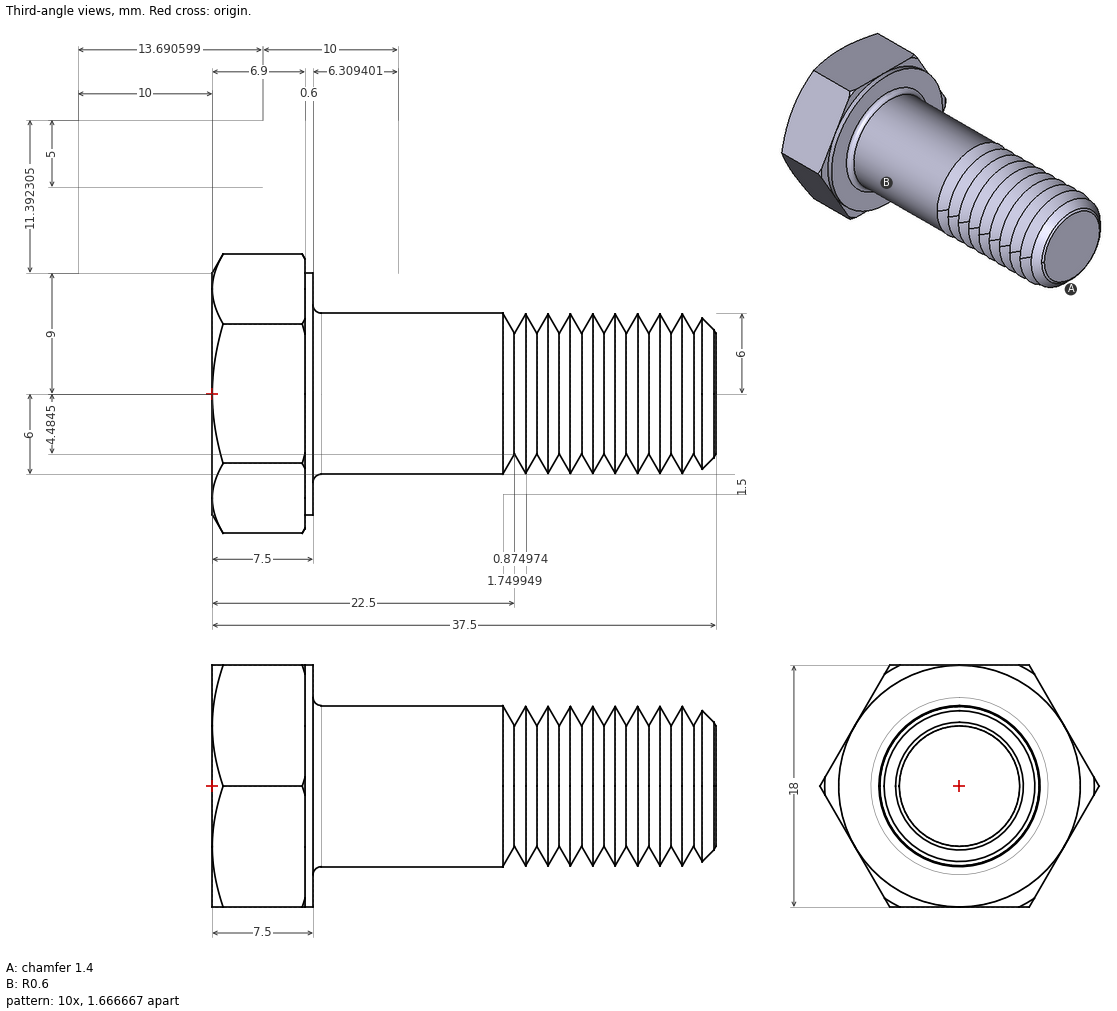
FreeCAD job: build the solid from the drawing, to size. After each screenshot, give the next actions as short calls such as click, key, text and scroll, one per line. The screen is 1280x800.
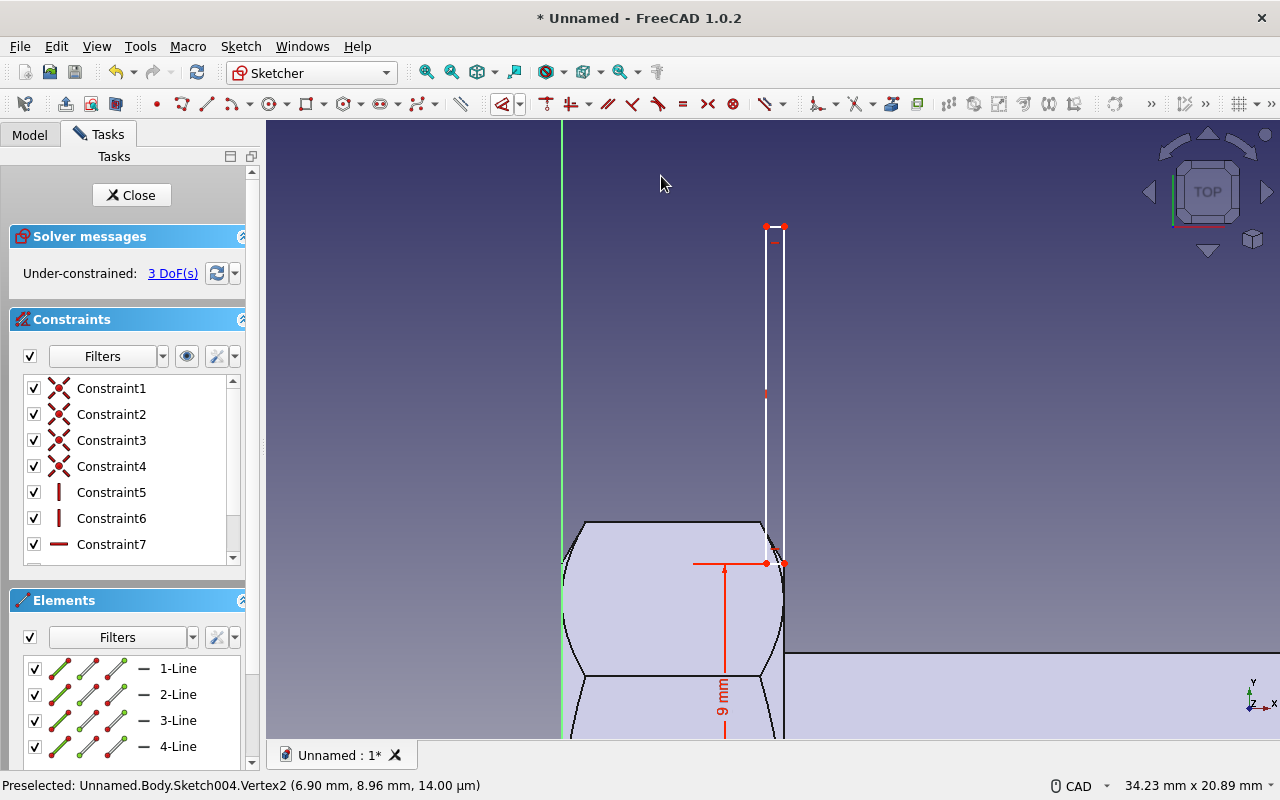
scroll(775, 564, up, 5)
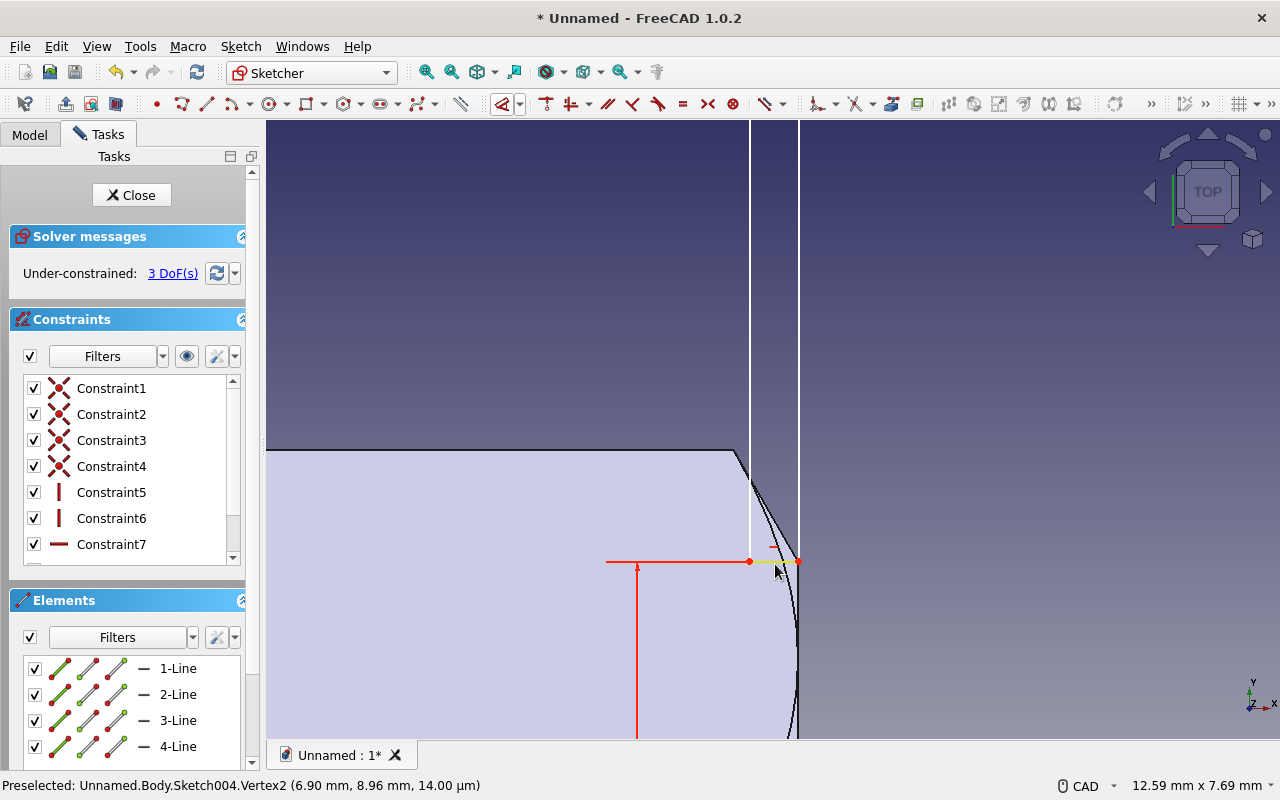
click(774, 562)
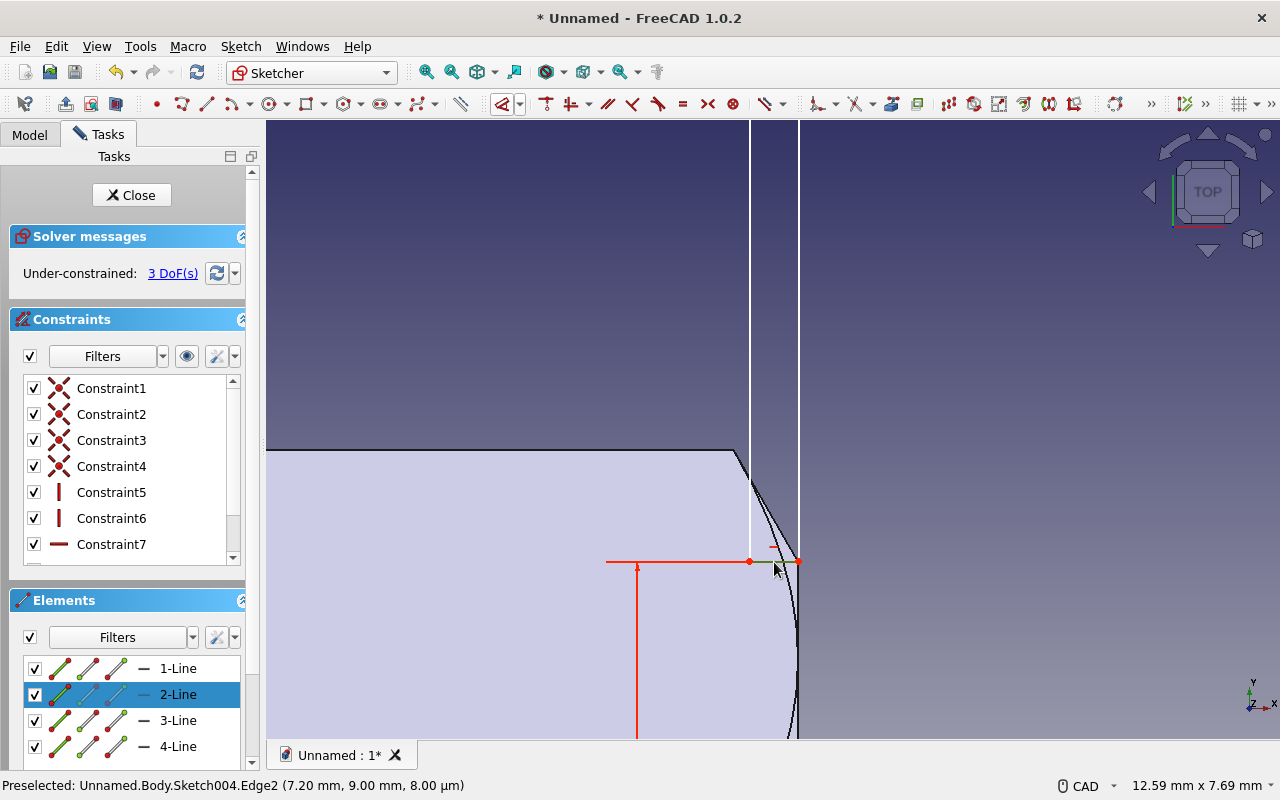
key(l)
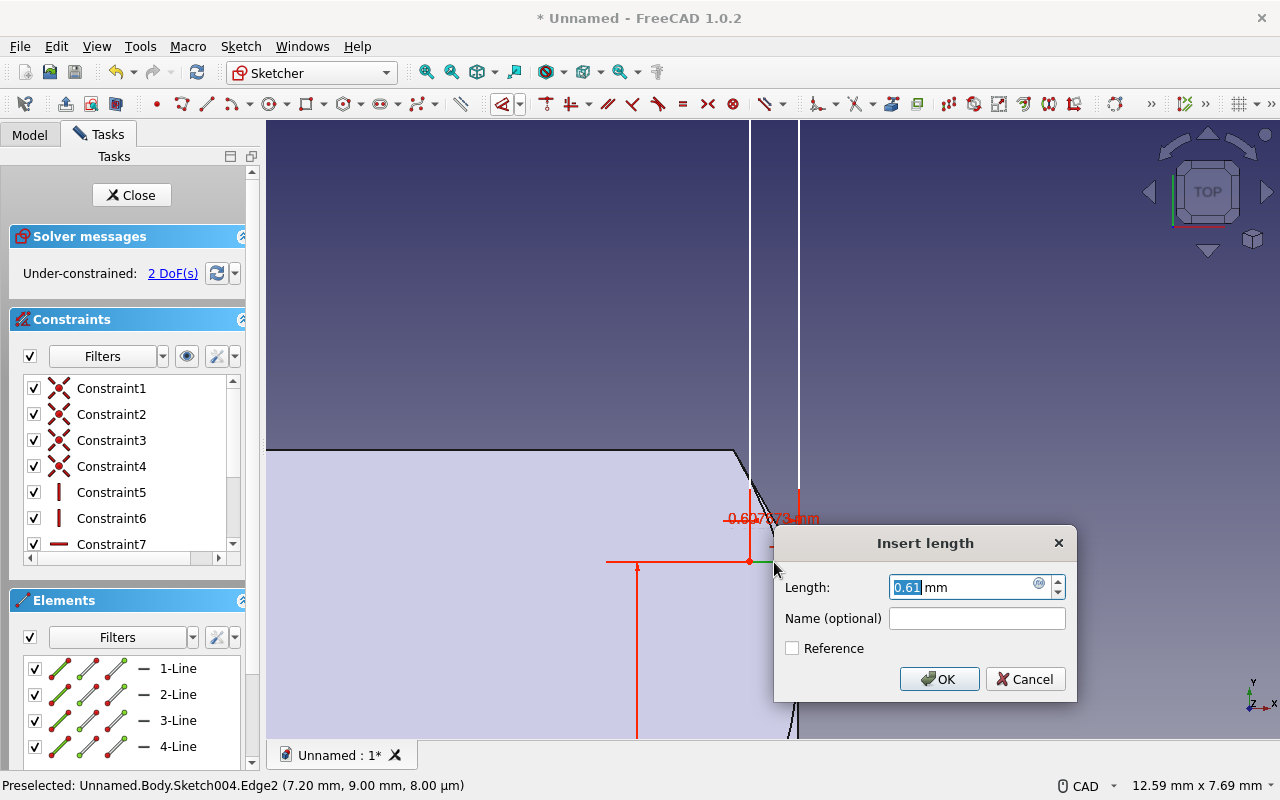
text(0.6)
key(Return)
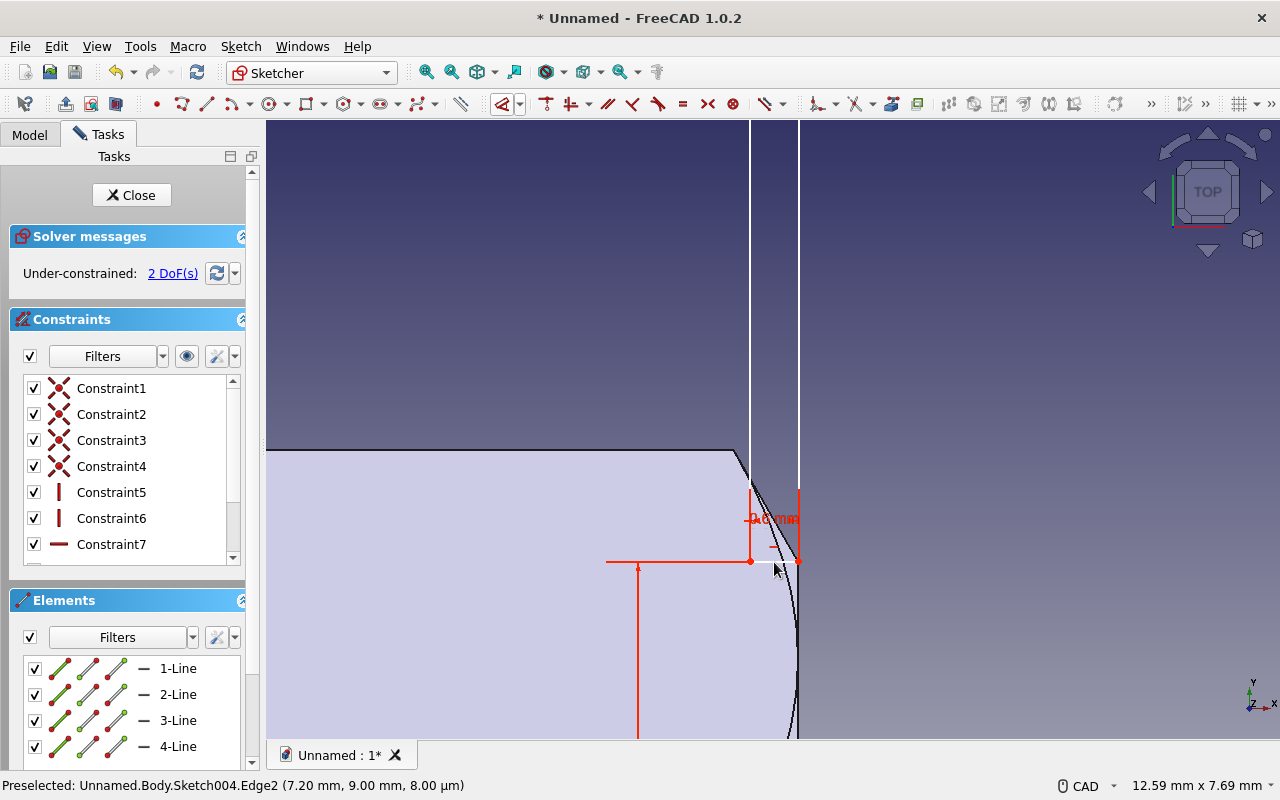
scroll(773, 418, down, 7)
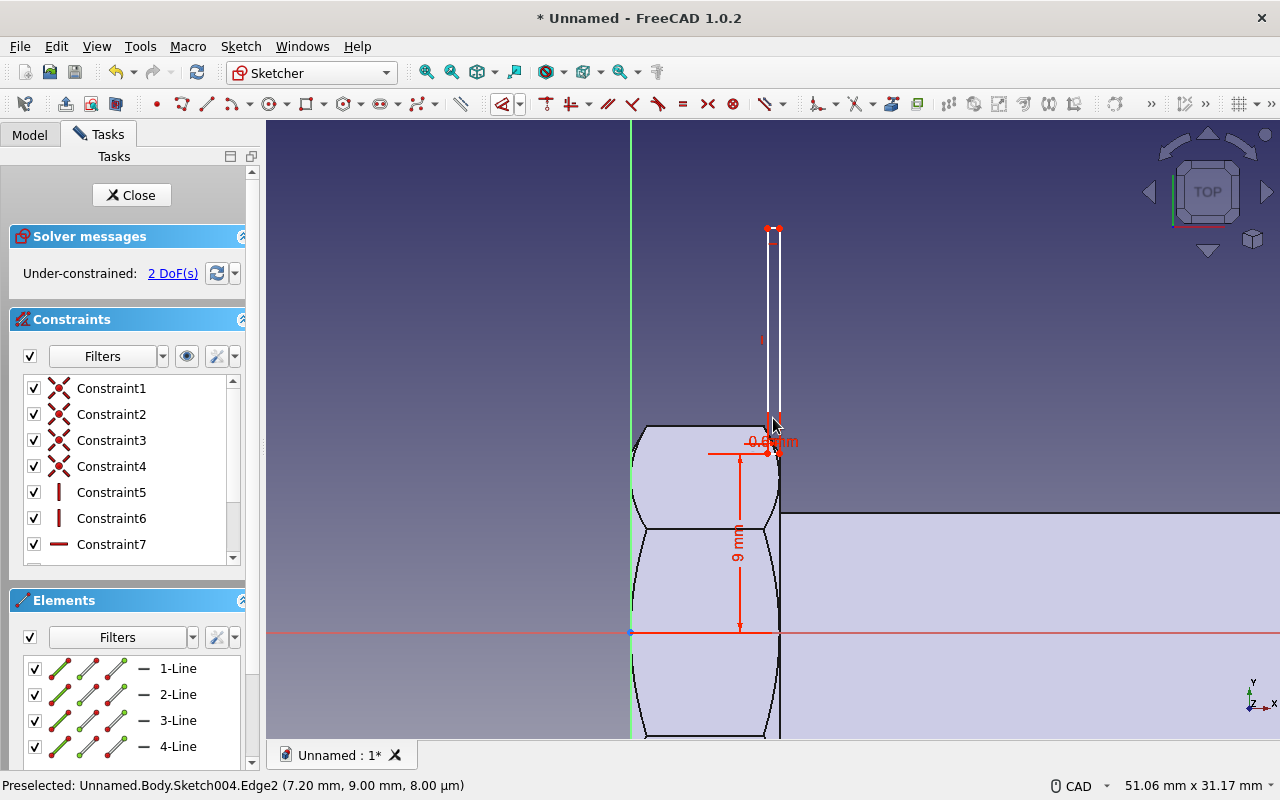
click(768, 228)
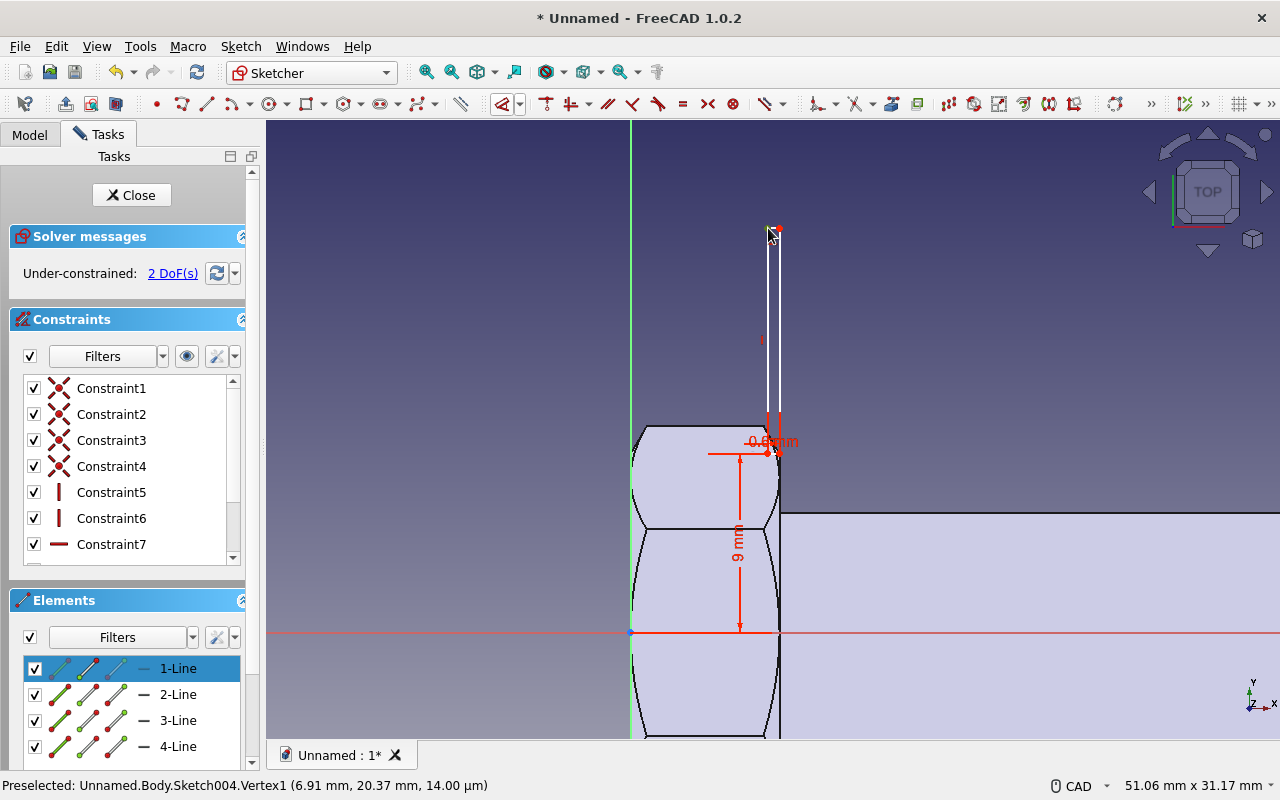
click(520, 104)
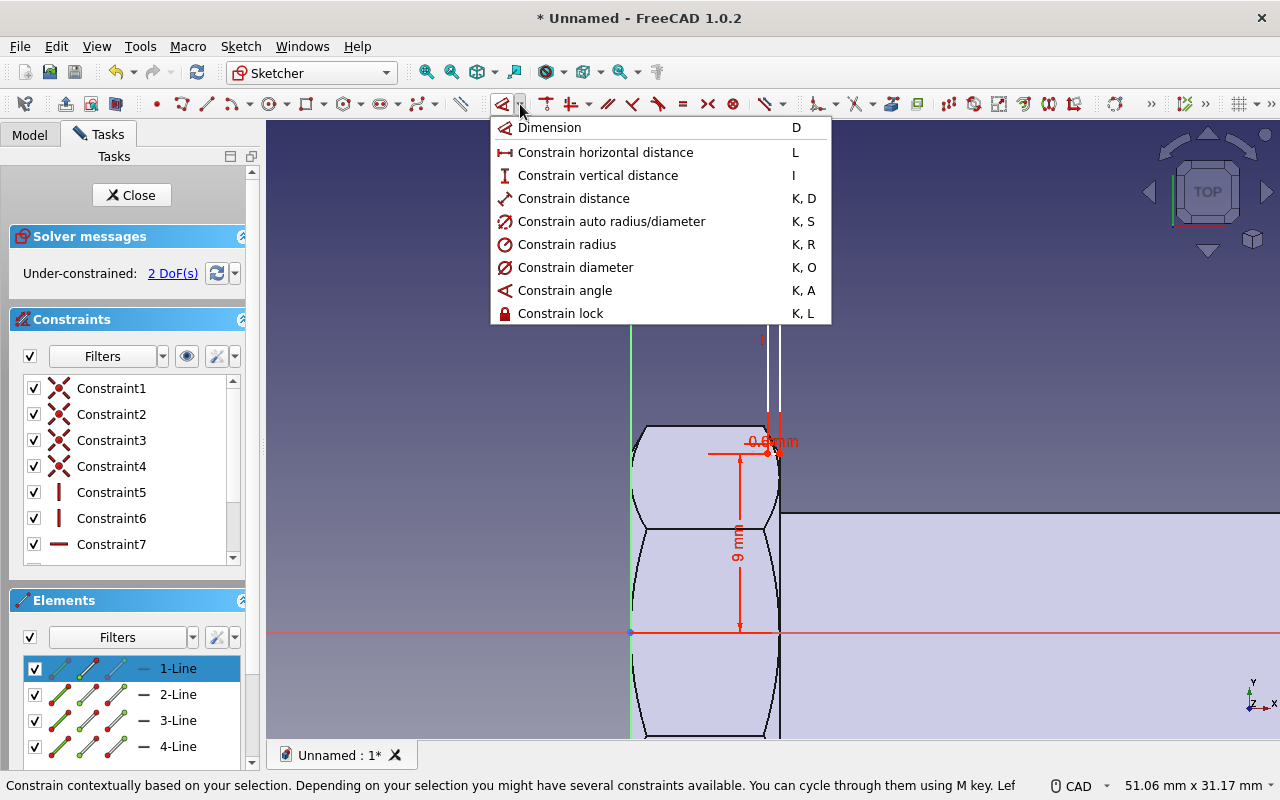
click(661, 152)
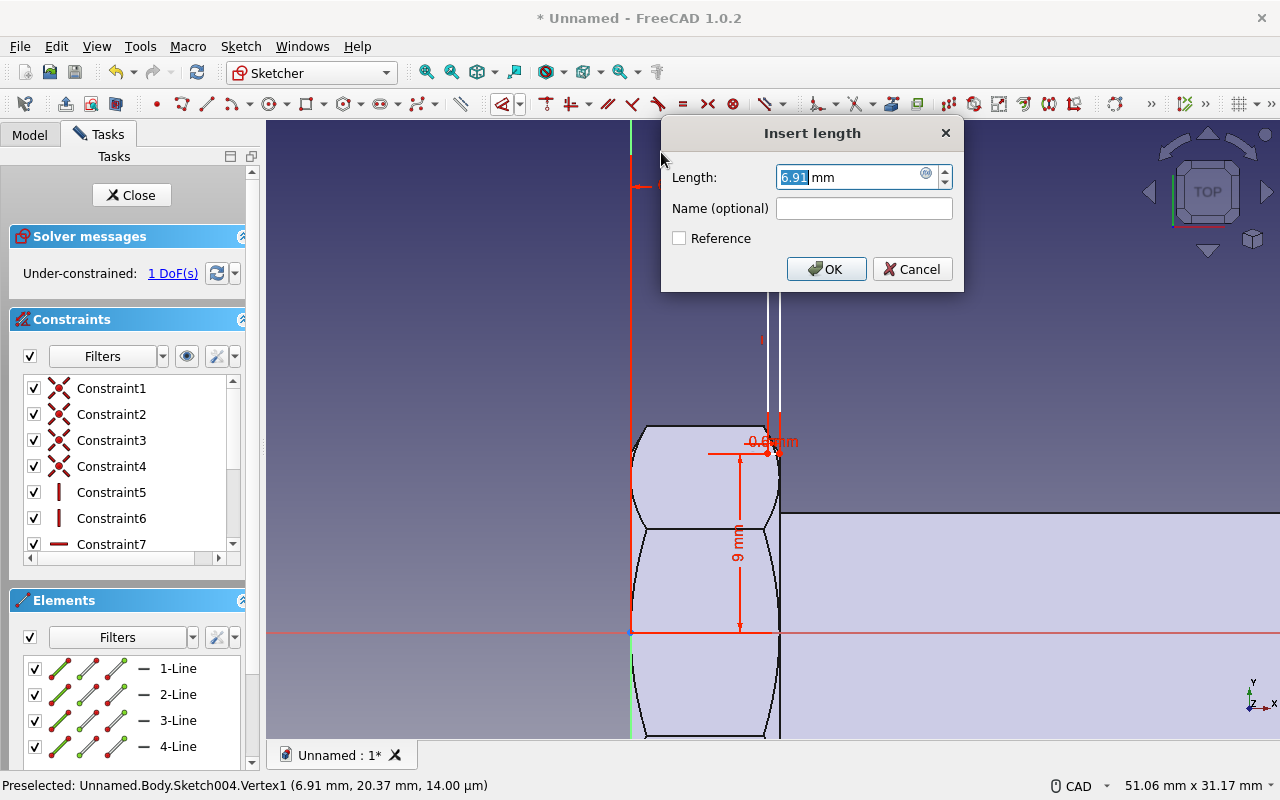
text(6.9)
key(Return)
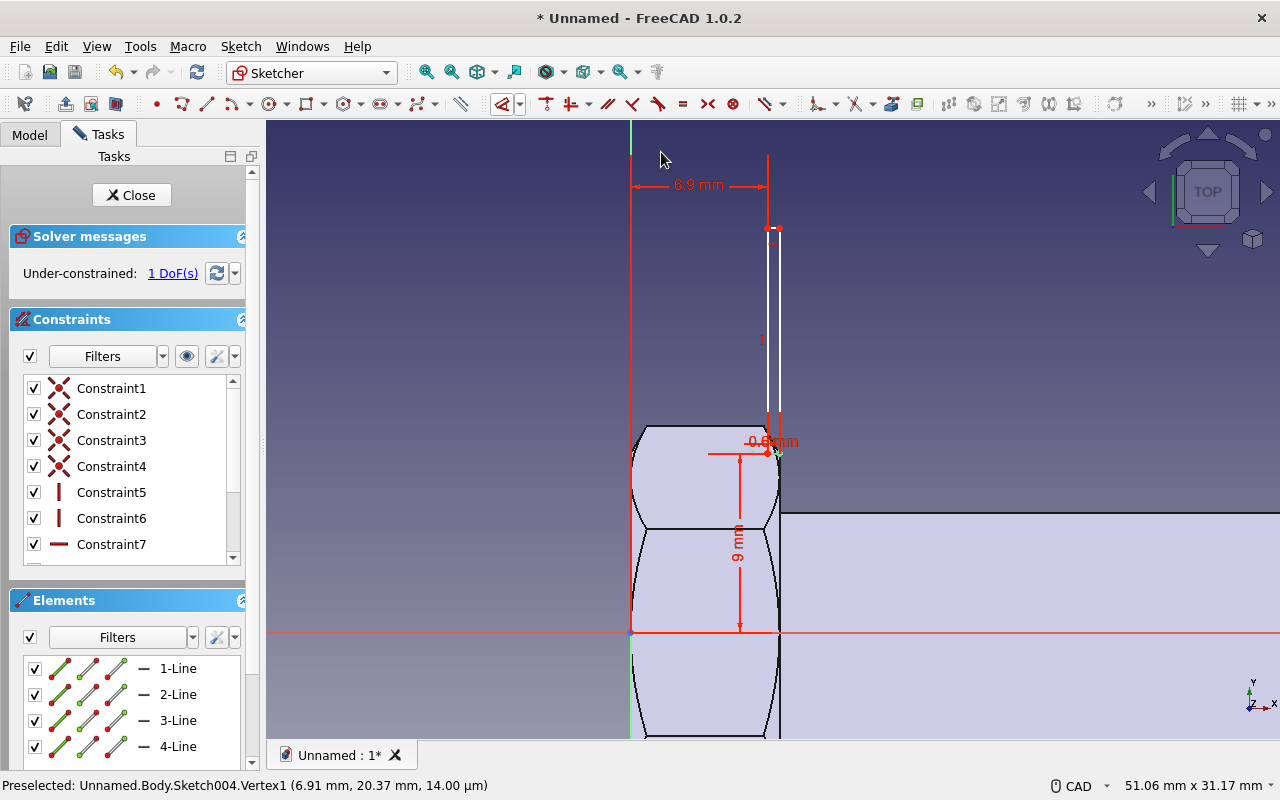
click(768, 296)